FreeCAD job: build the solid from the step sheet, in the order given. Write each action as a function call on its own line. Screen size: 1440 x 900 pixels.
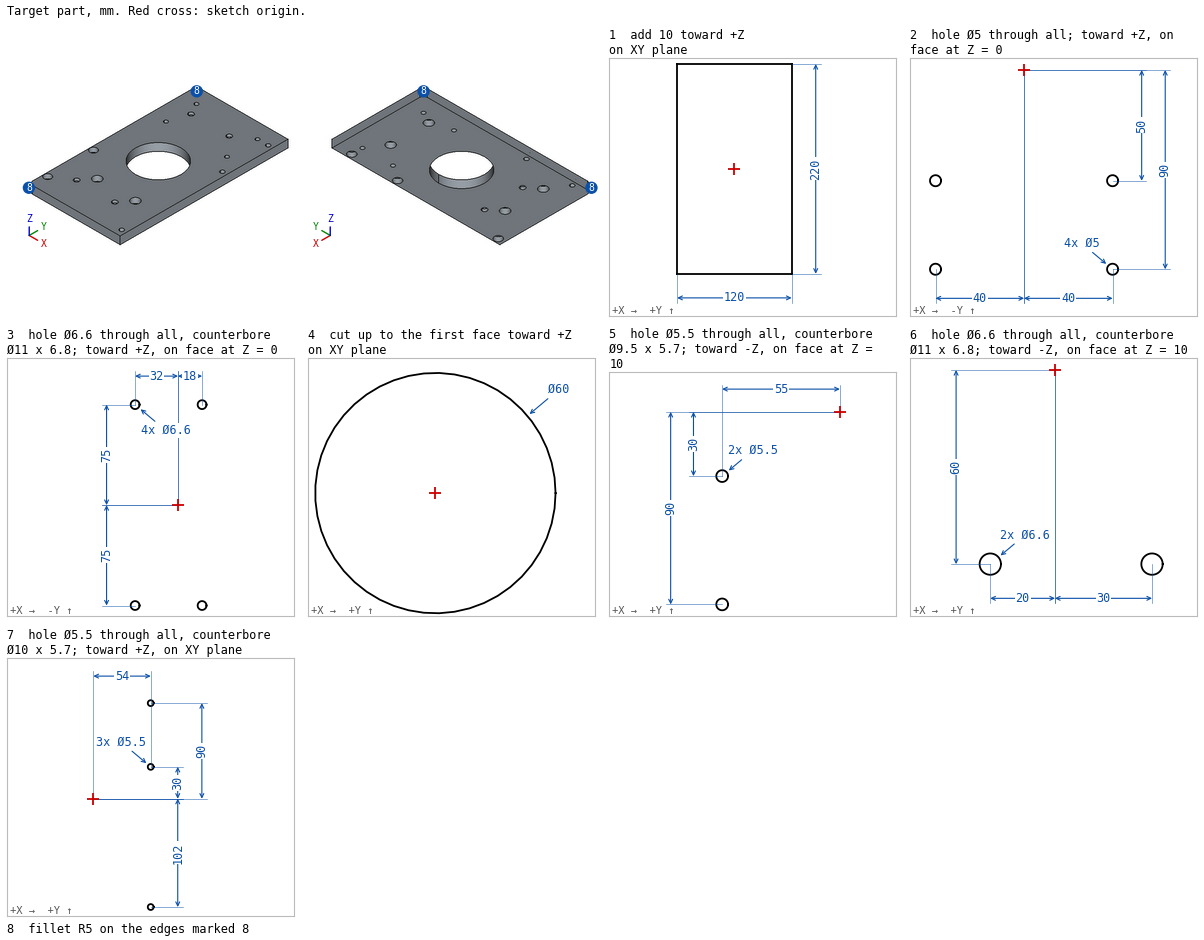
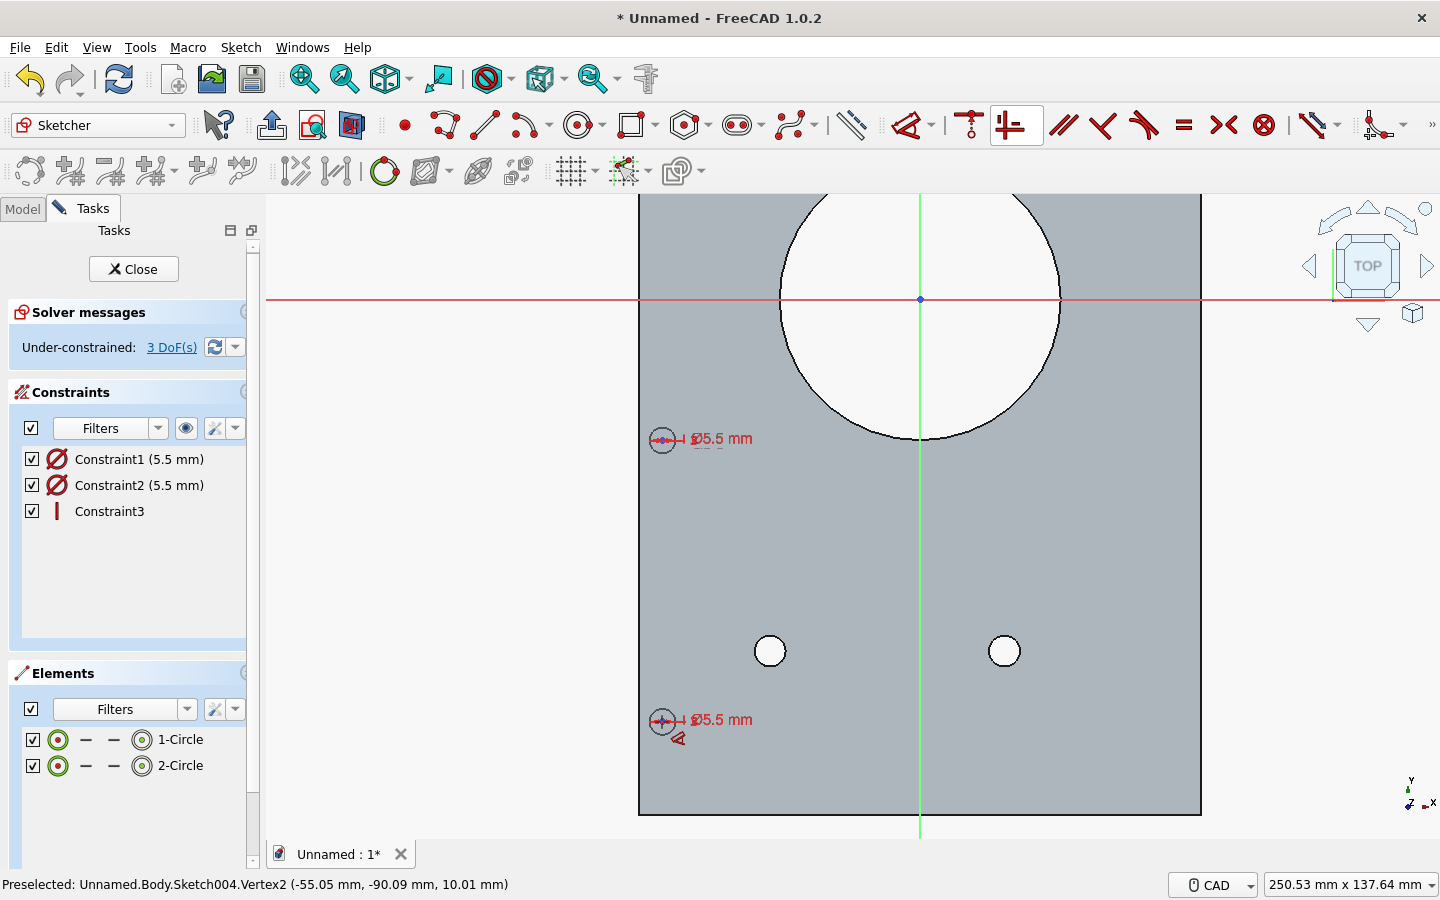
click(663, 441)
click(791, 266)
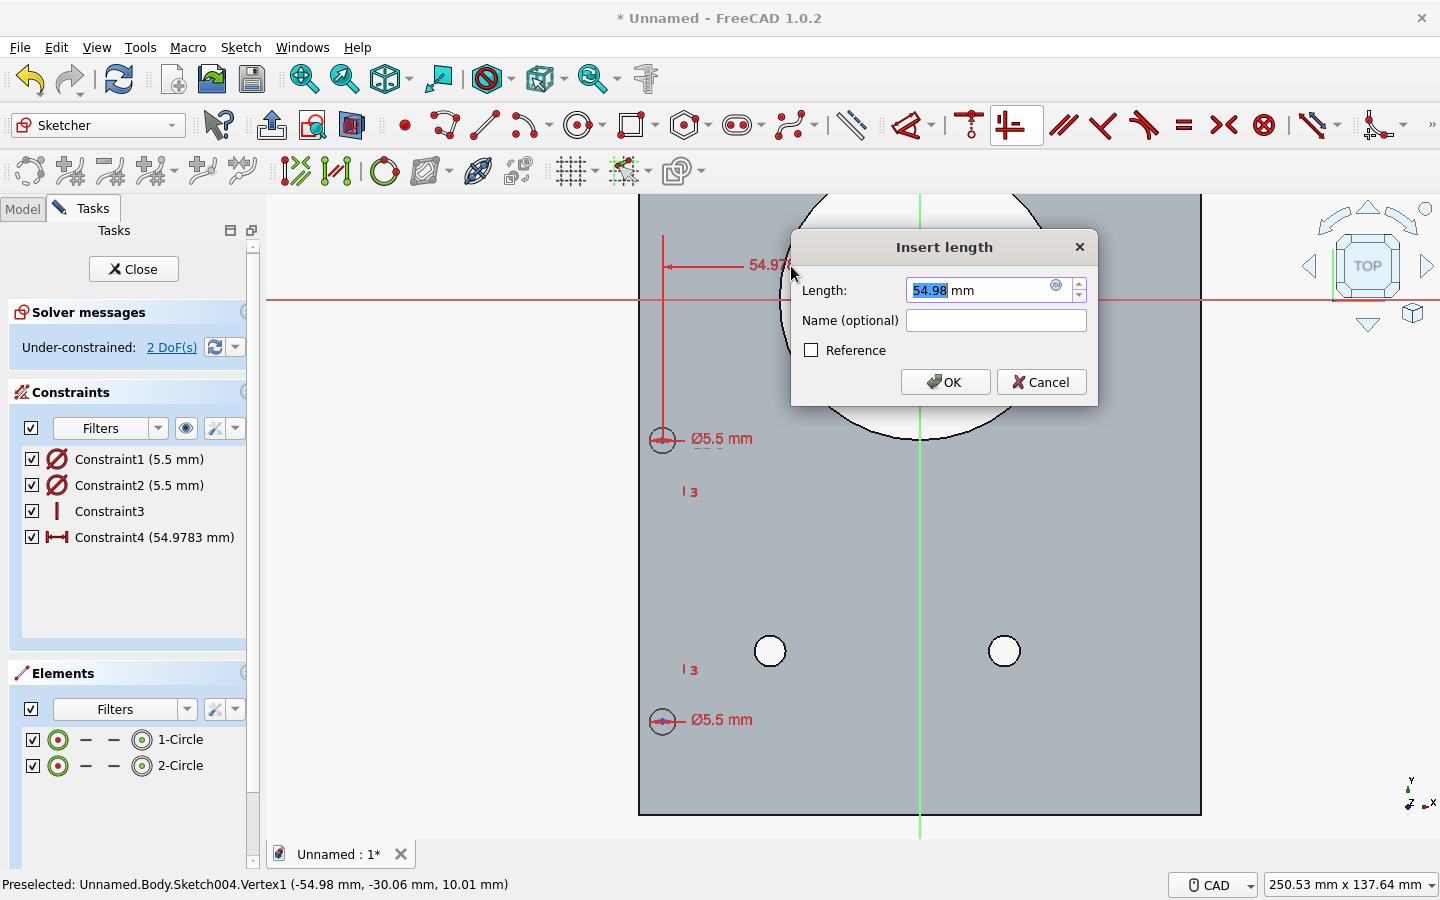
text(55)
key(Return)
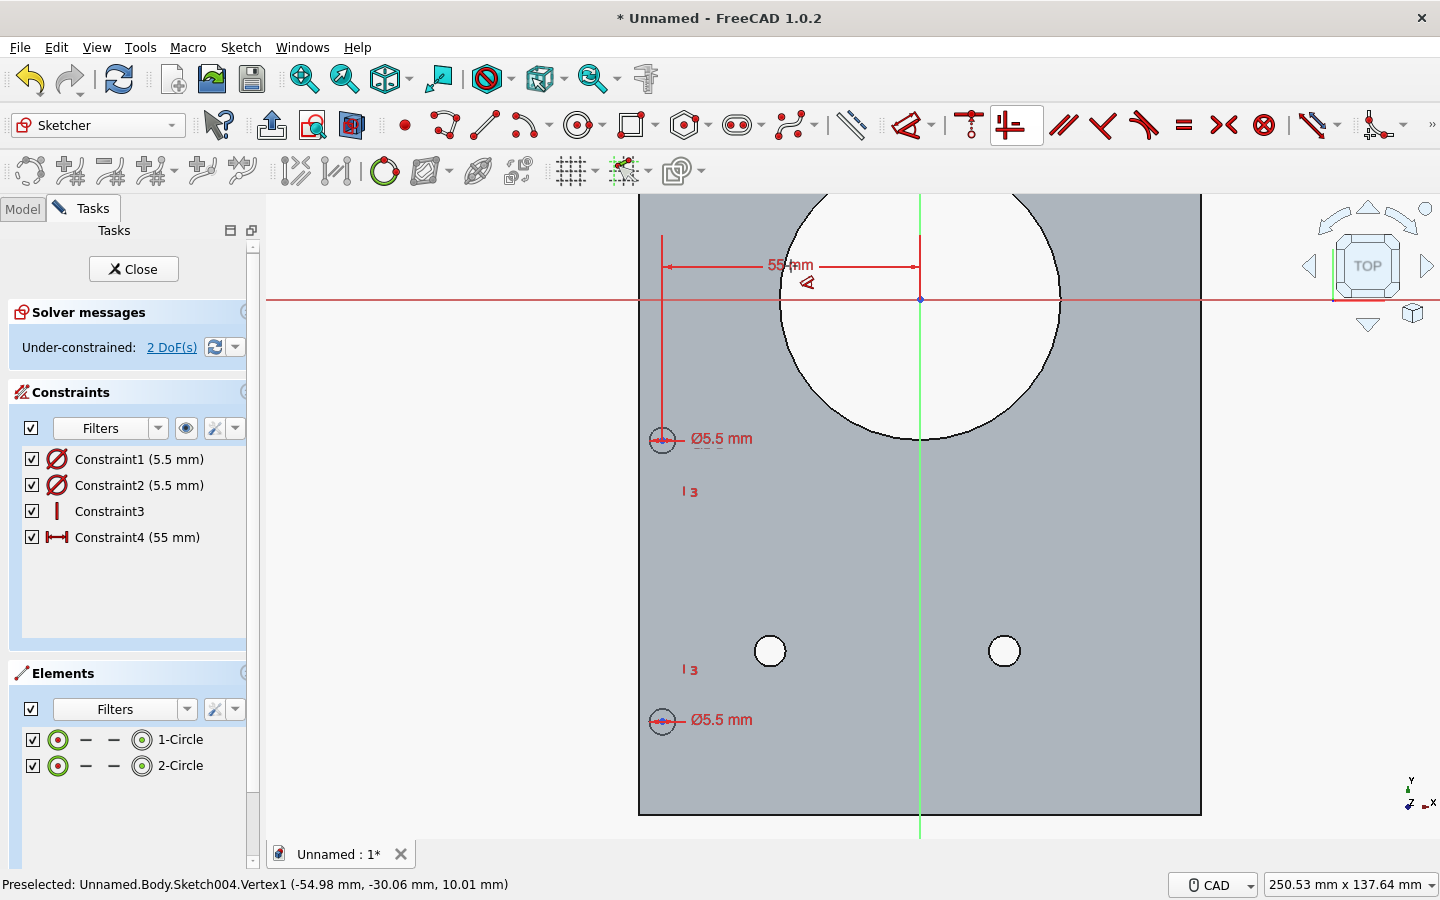
click(662, 441)
click(954, 370)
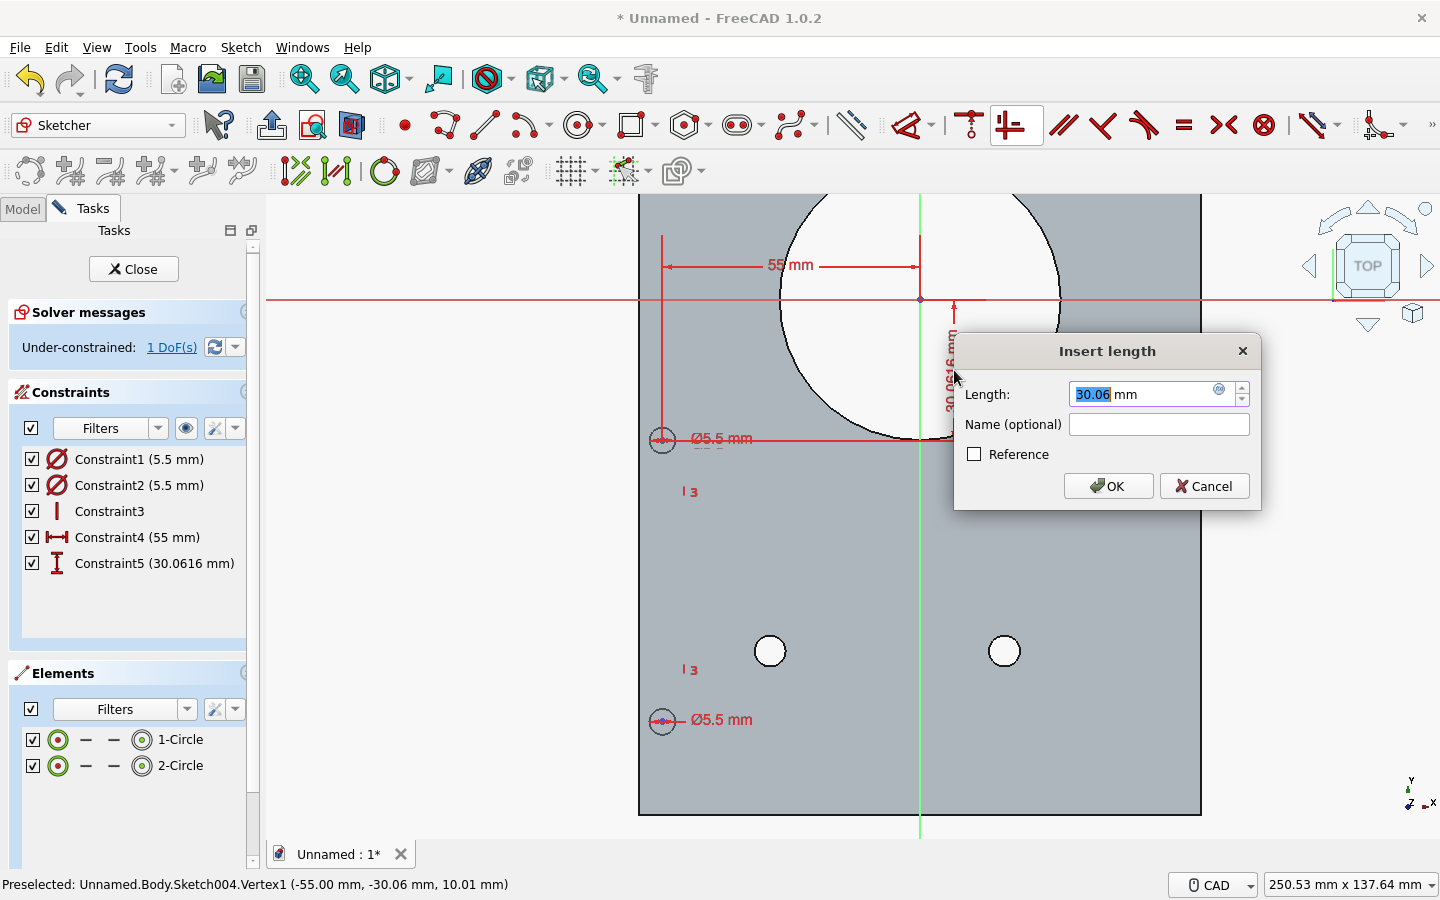
text(30)
key(Return)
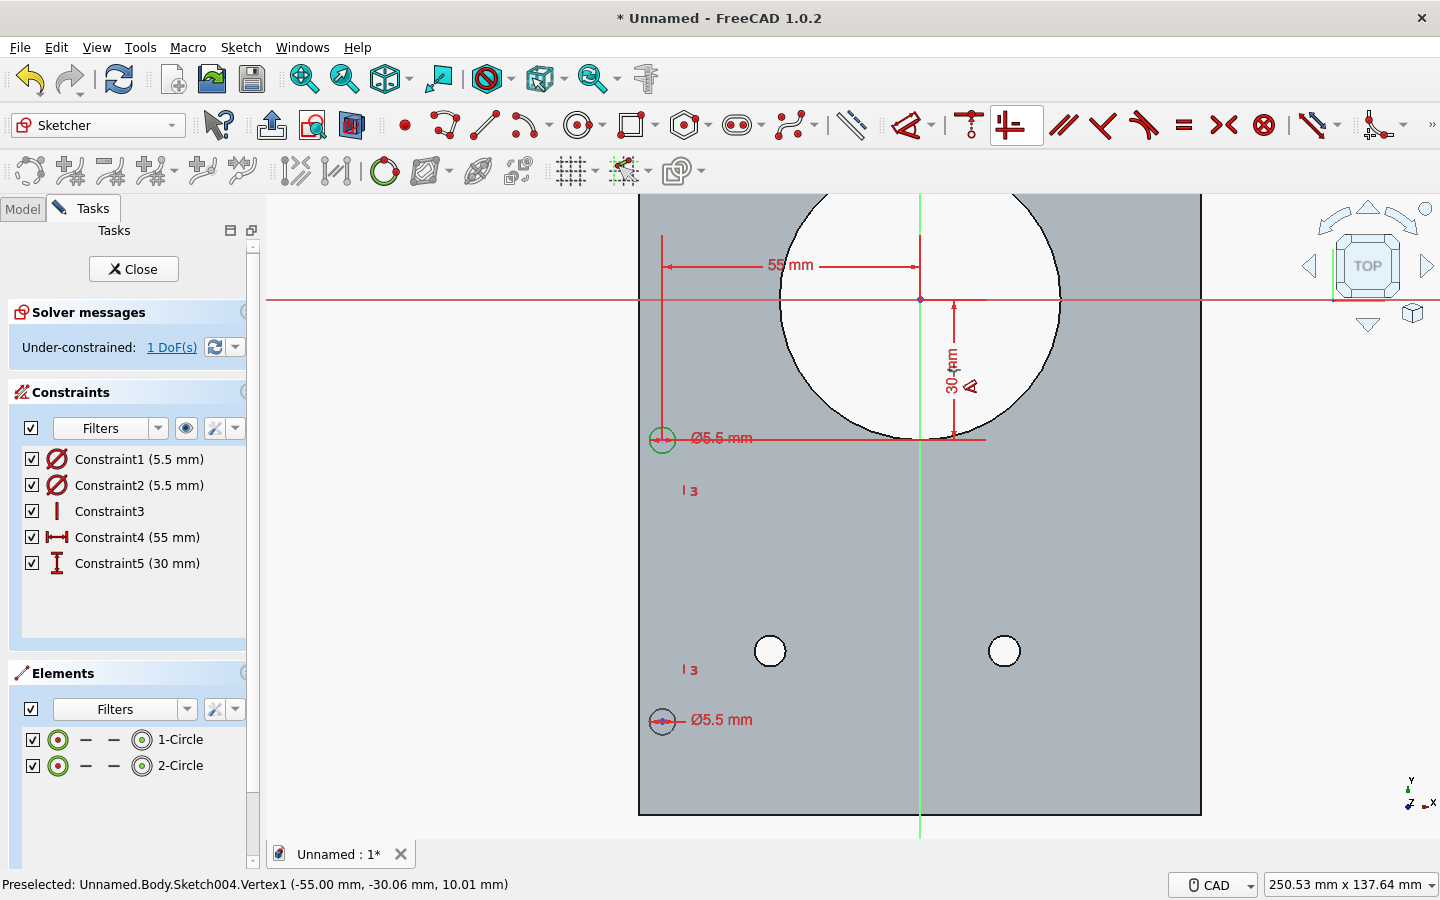
click(662, 722)
click(954, 511)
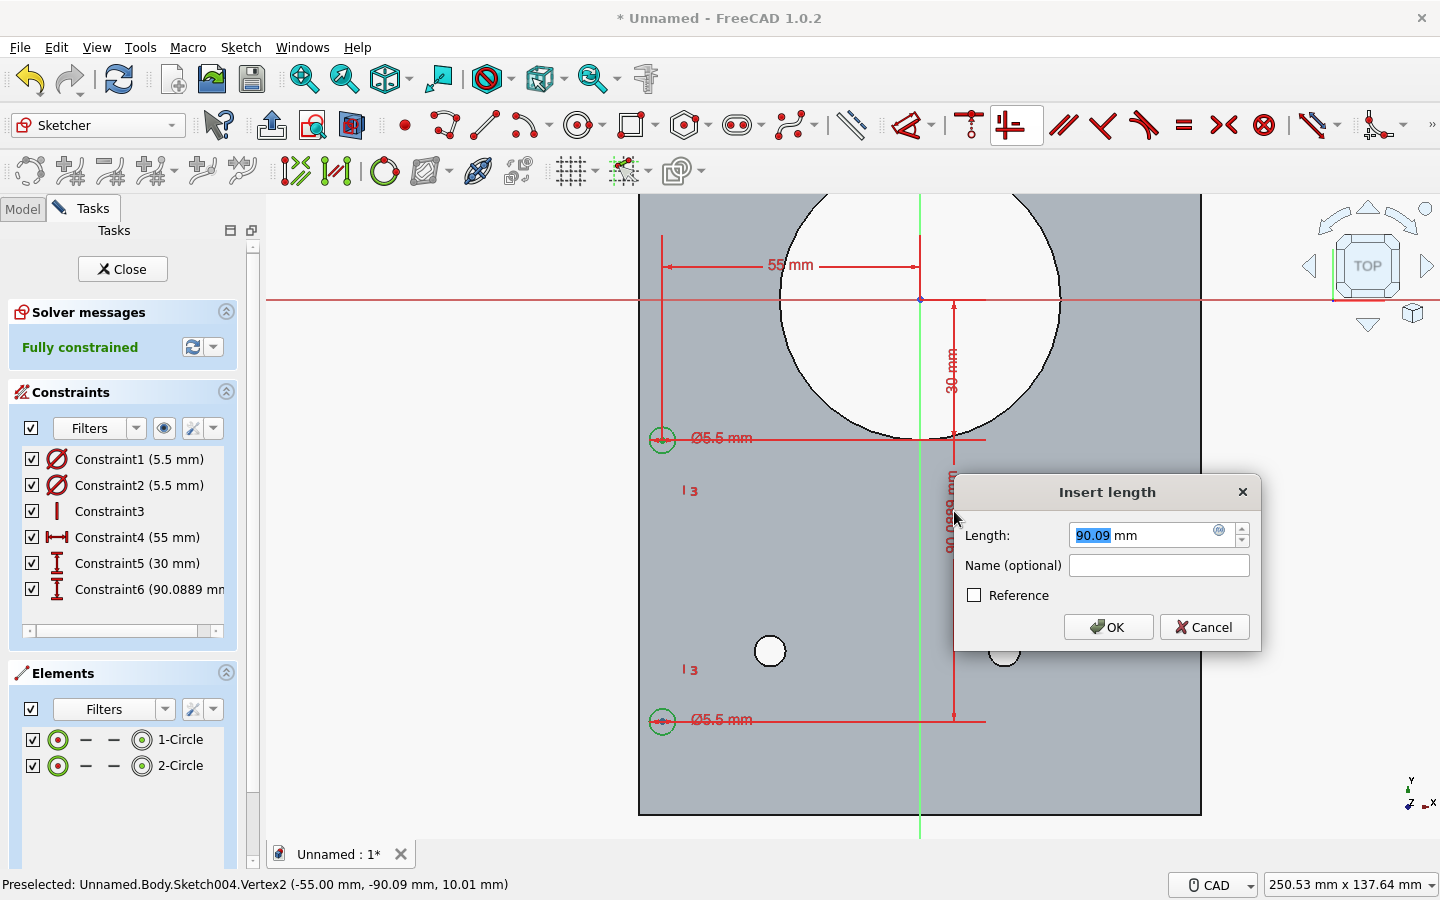
text(90)
key(Return)
key(Escape)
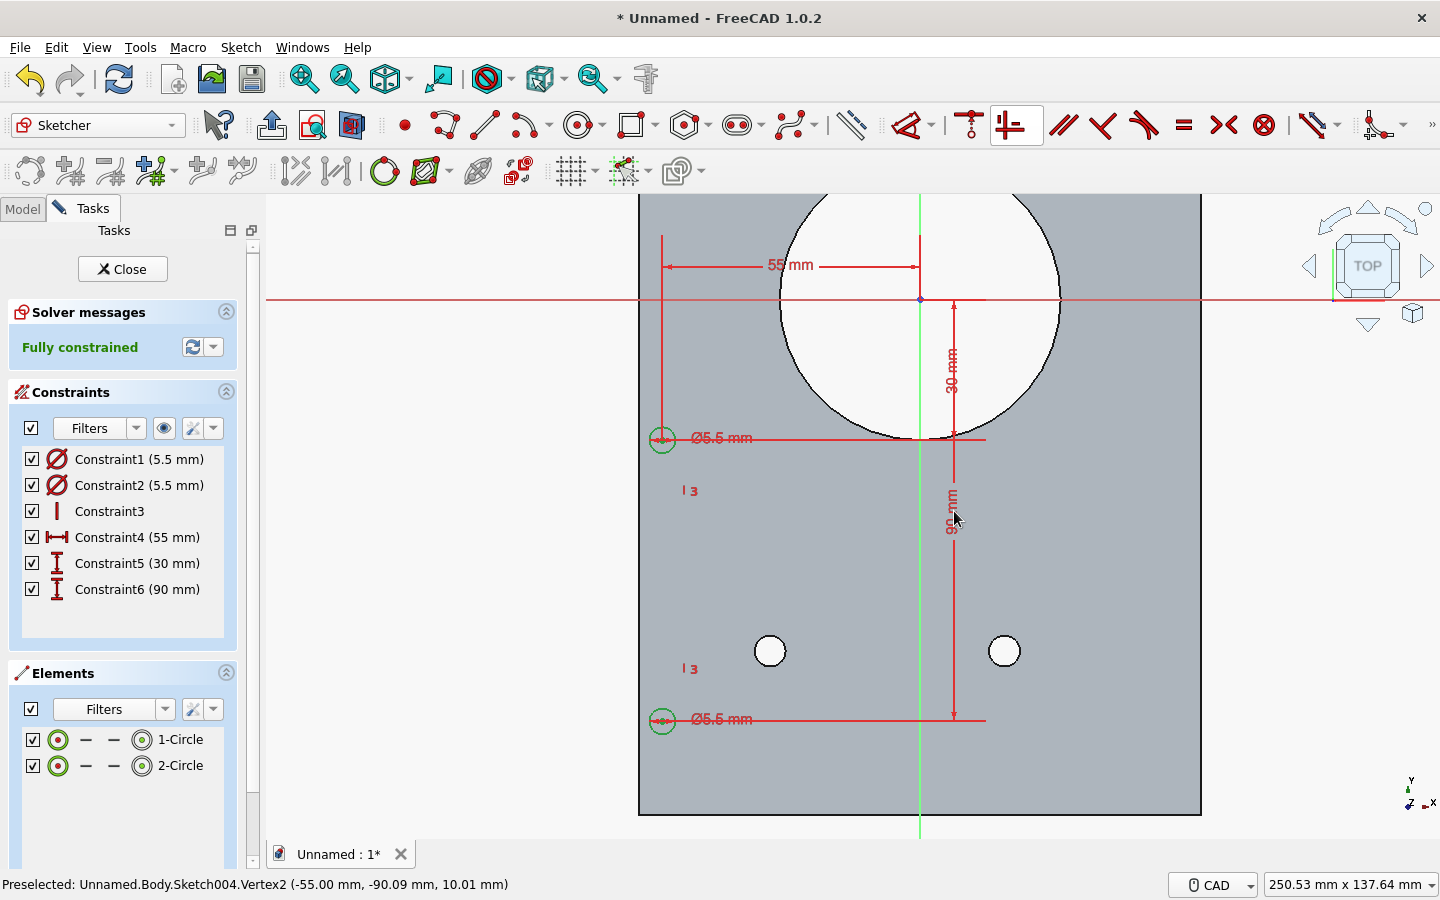
click(123, 269)